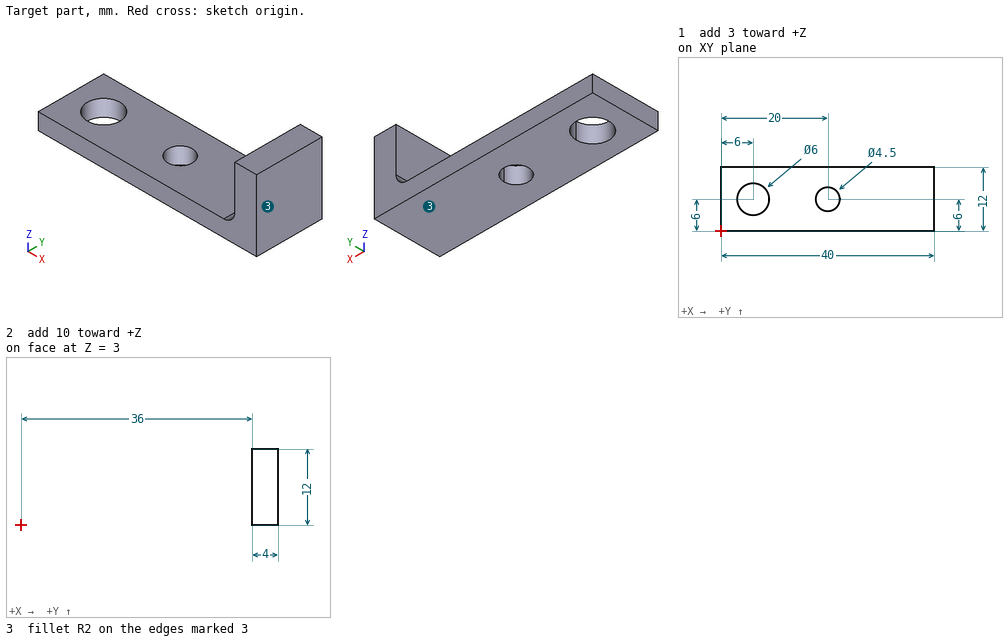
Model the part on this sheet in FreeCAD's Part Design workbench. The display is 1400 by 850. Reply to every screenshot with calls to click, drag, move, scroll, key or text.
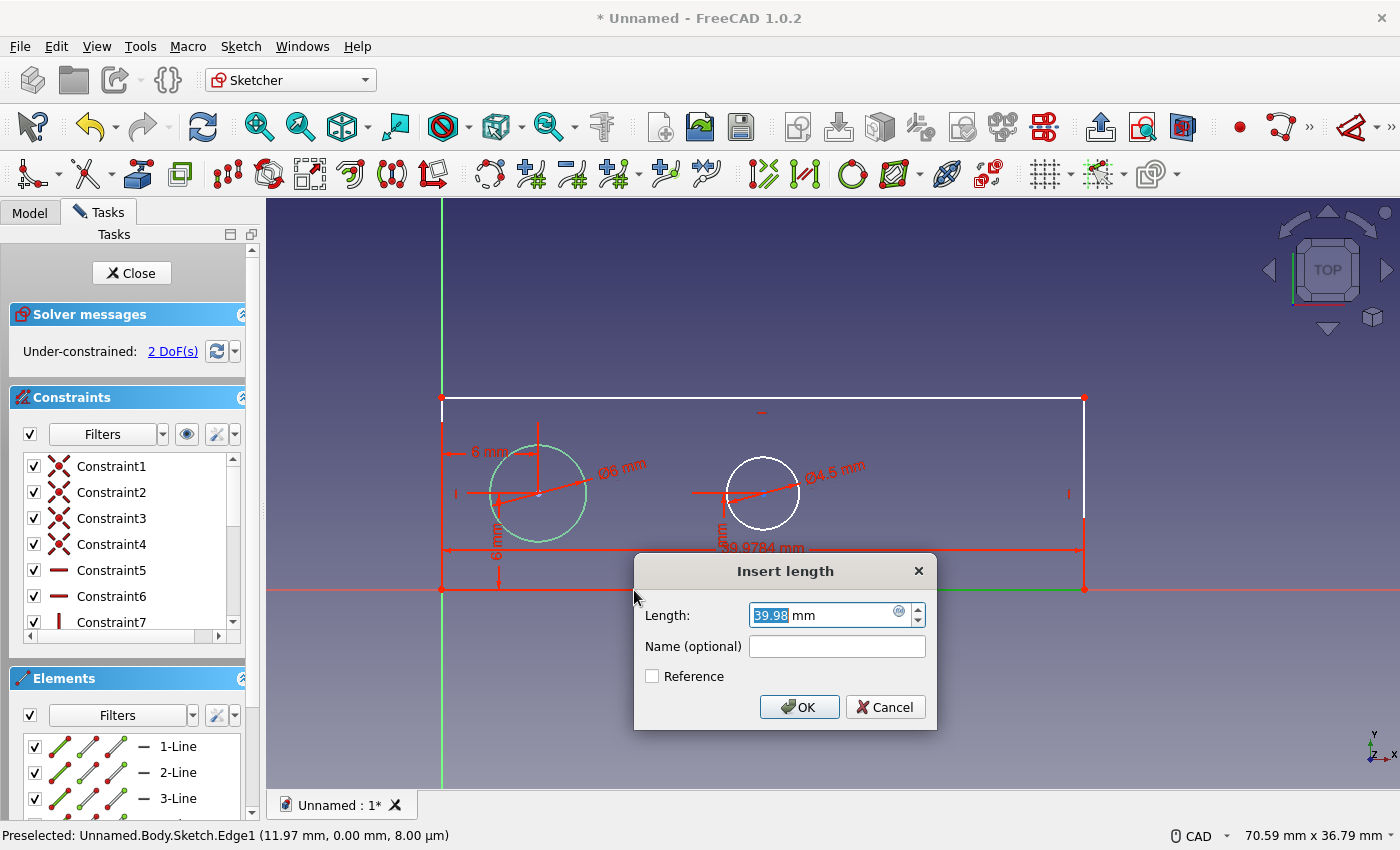
text(40)
key(Return)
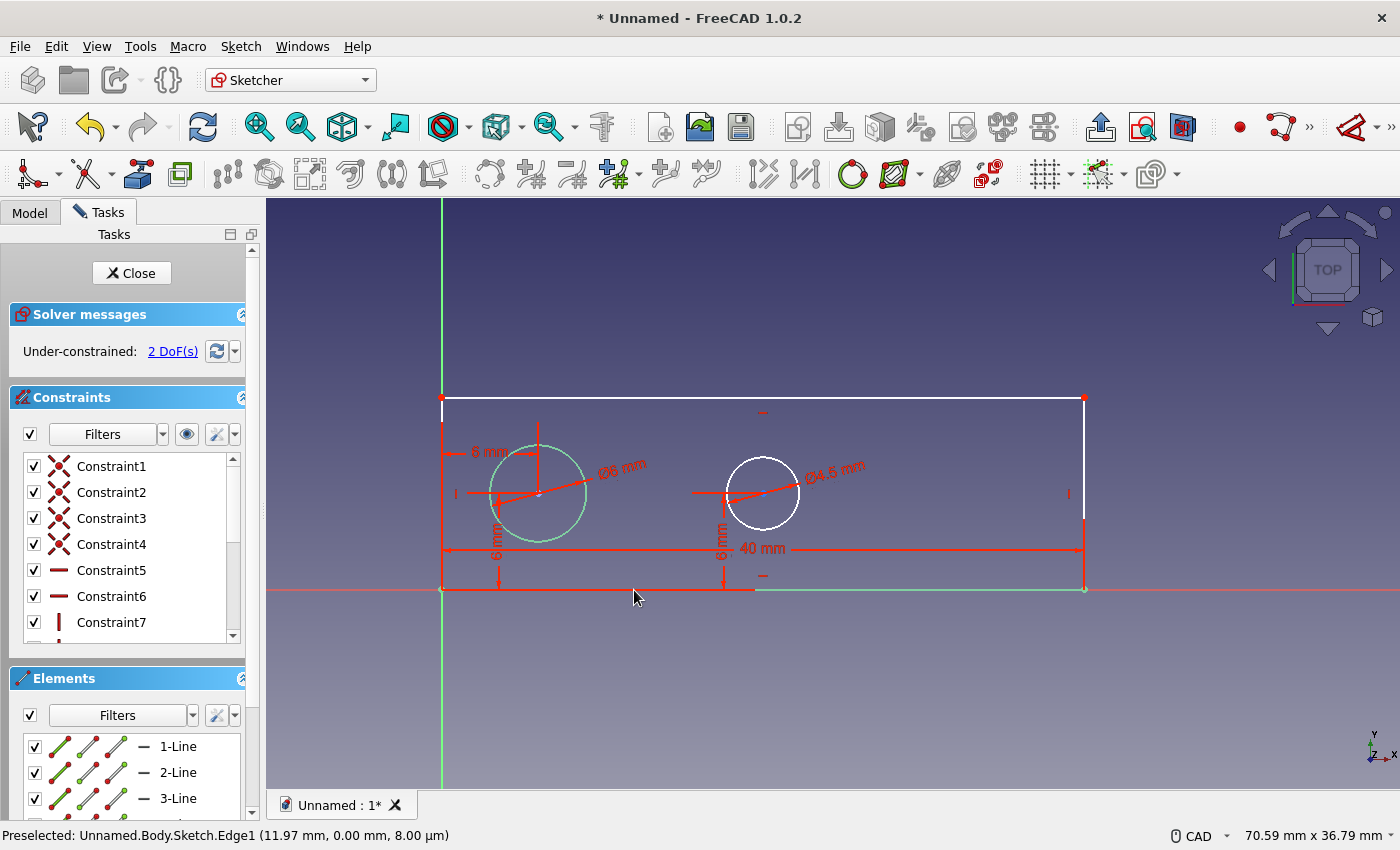
click(1084, 532)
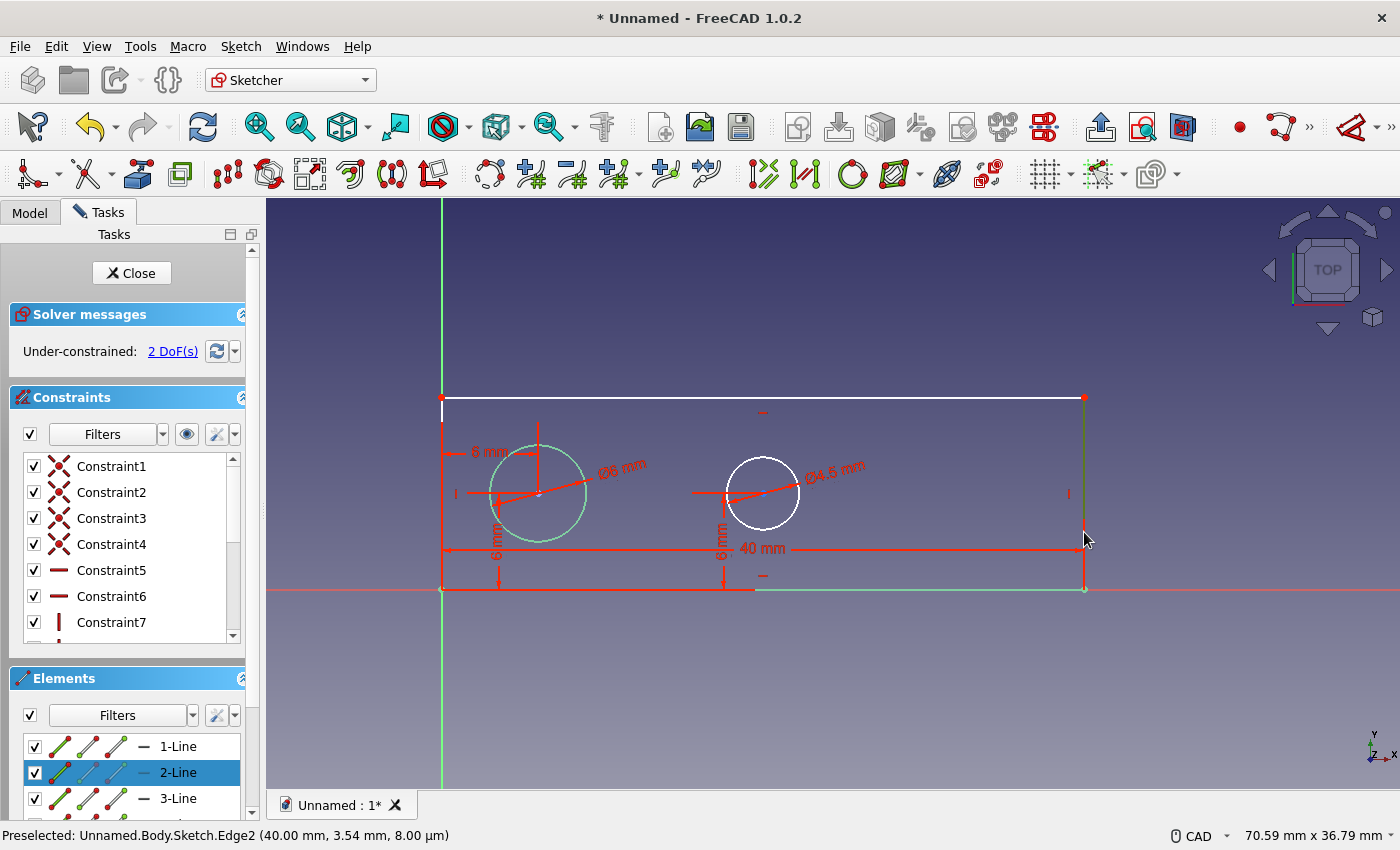
click(1376, 128)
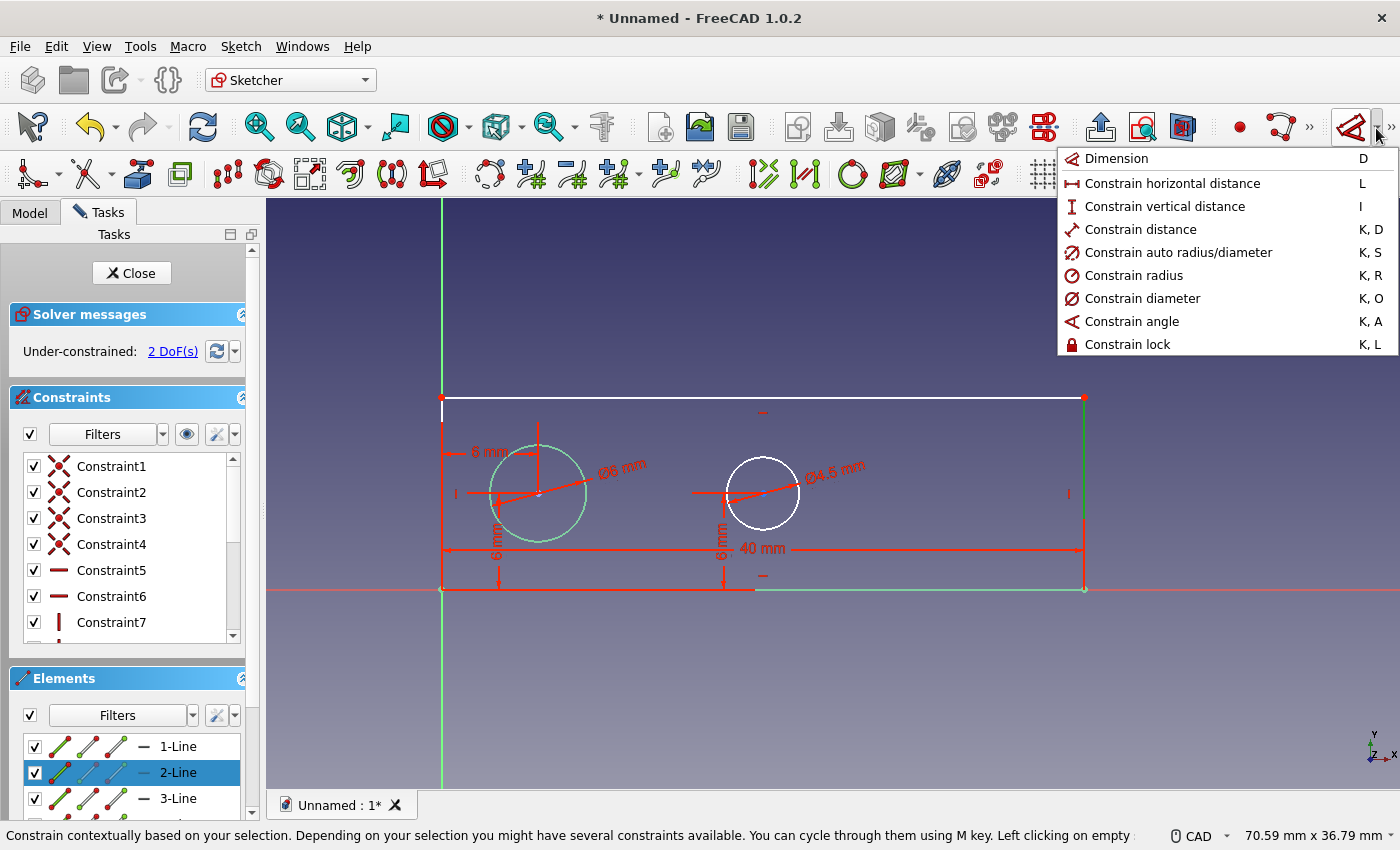
click(1228, 206)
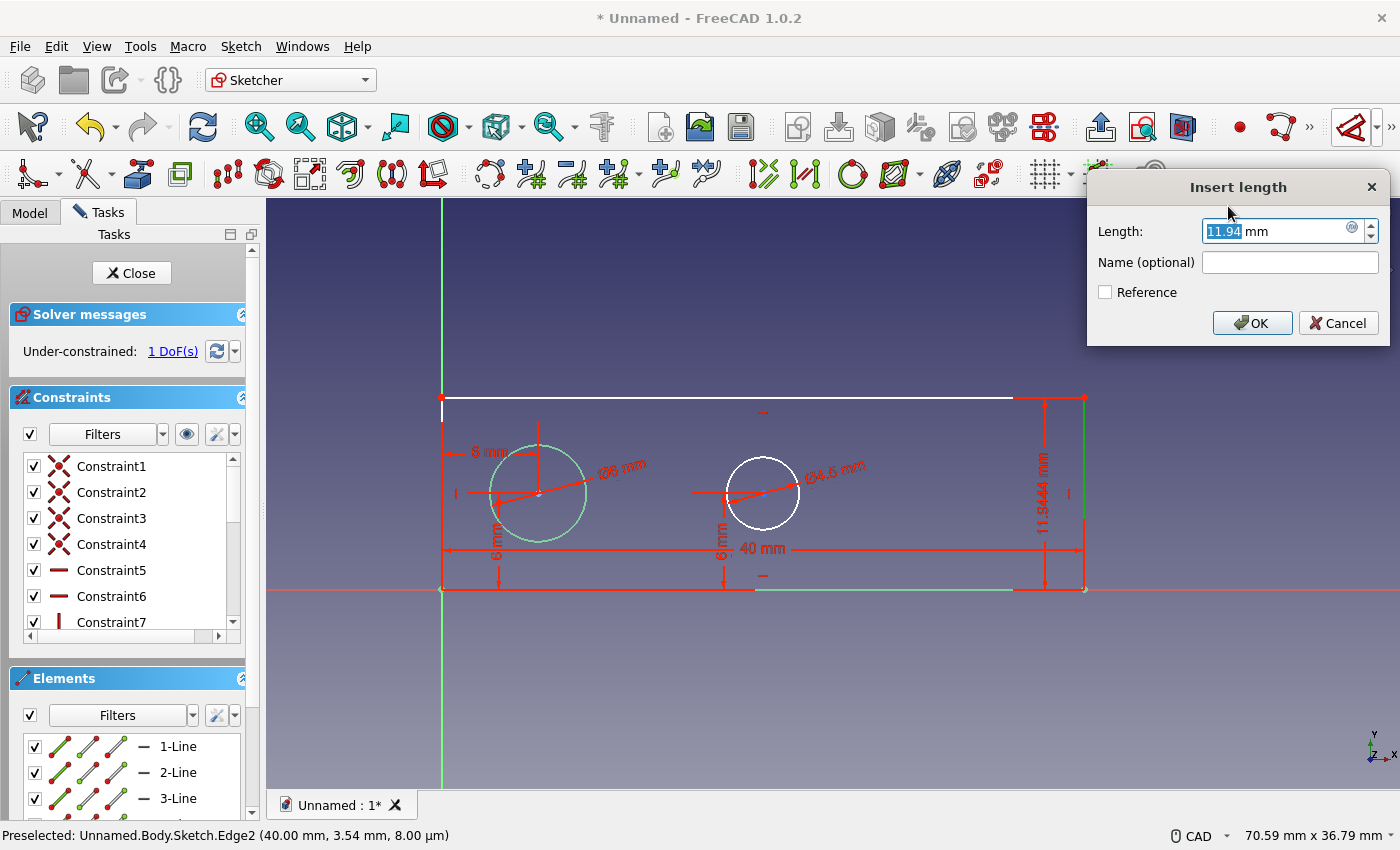
text(12)
key(Return)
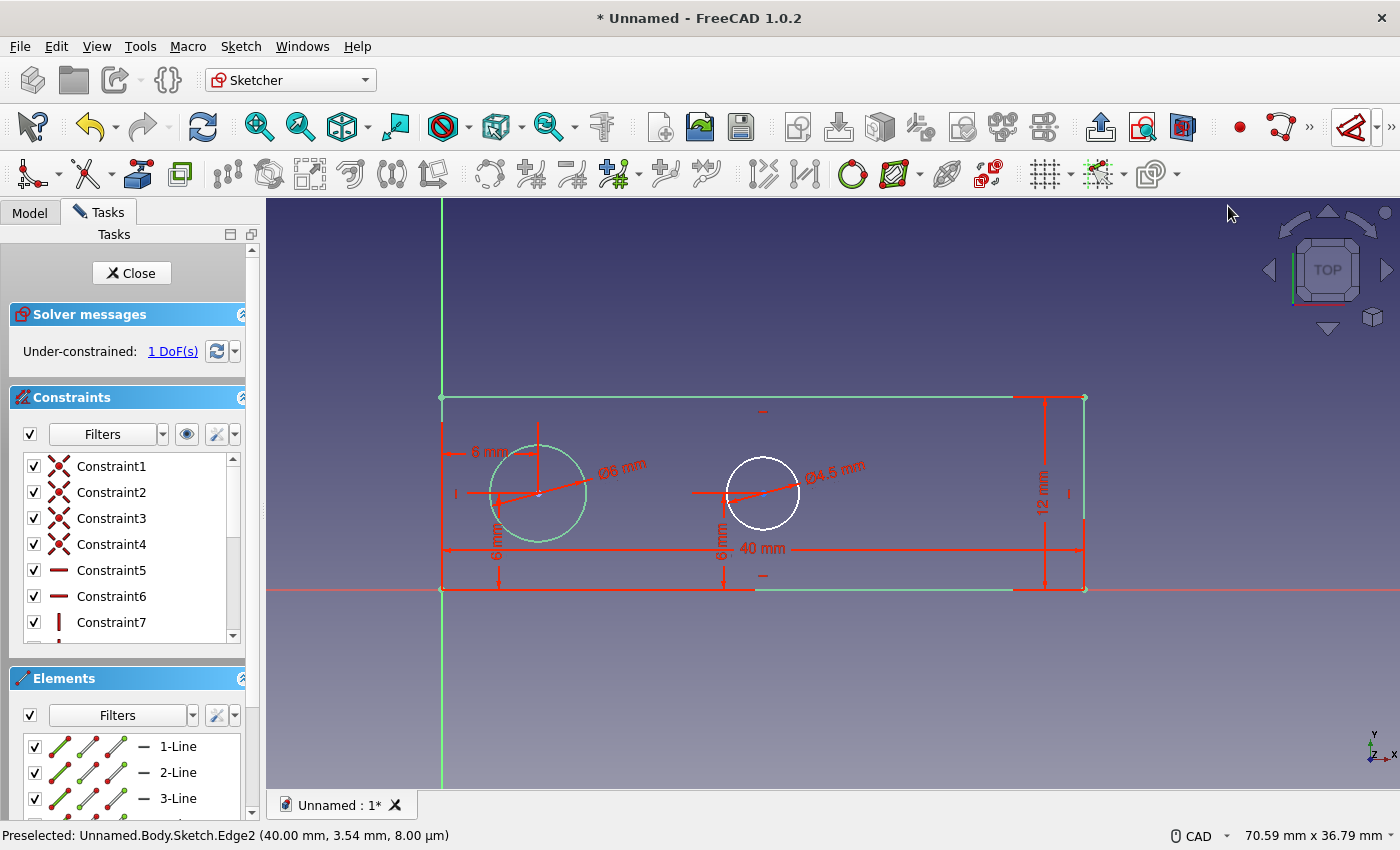
click(763, 493)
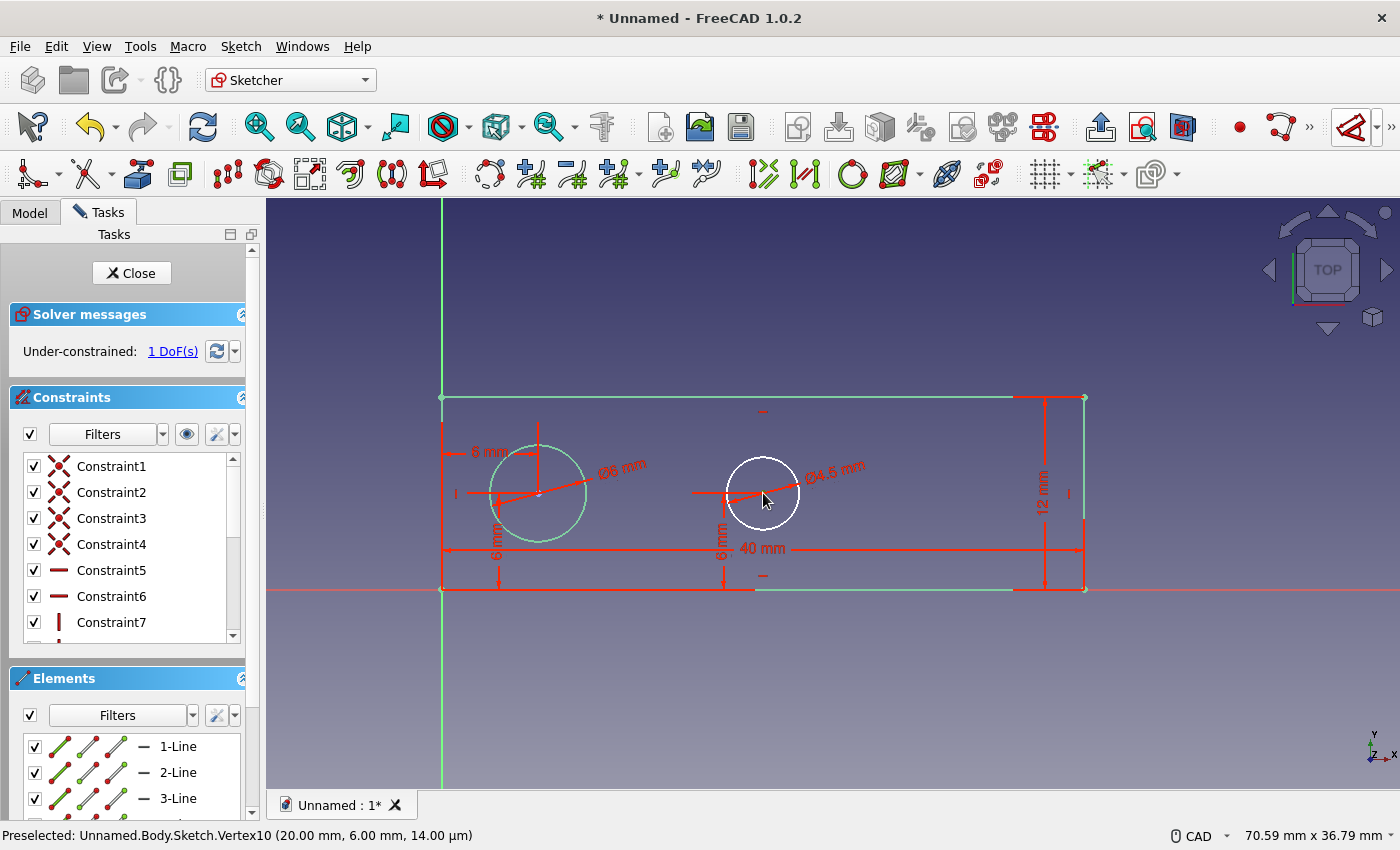
click(1376, 128)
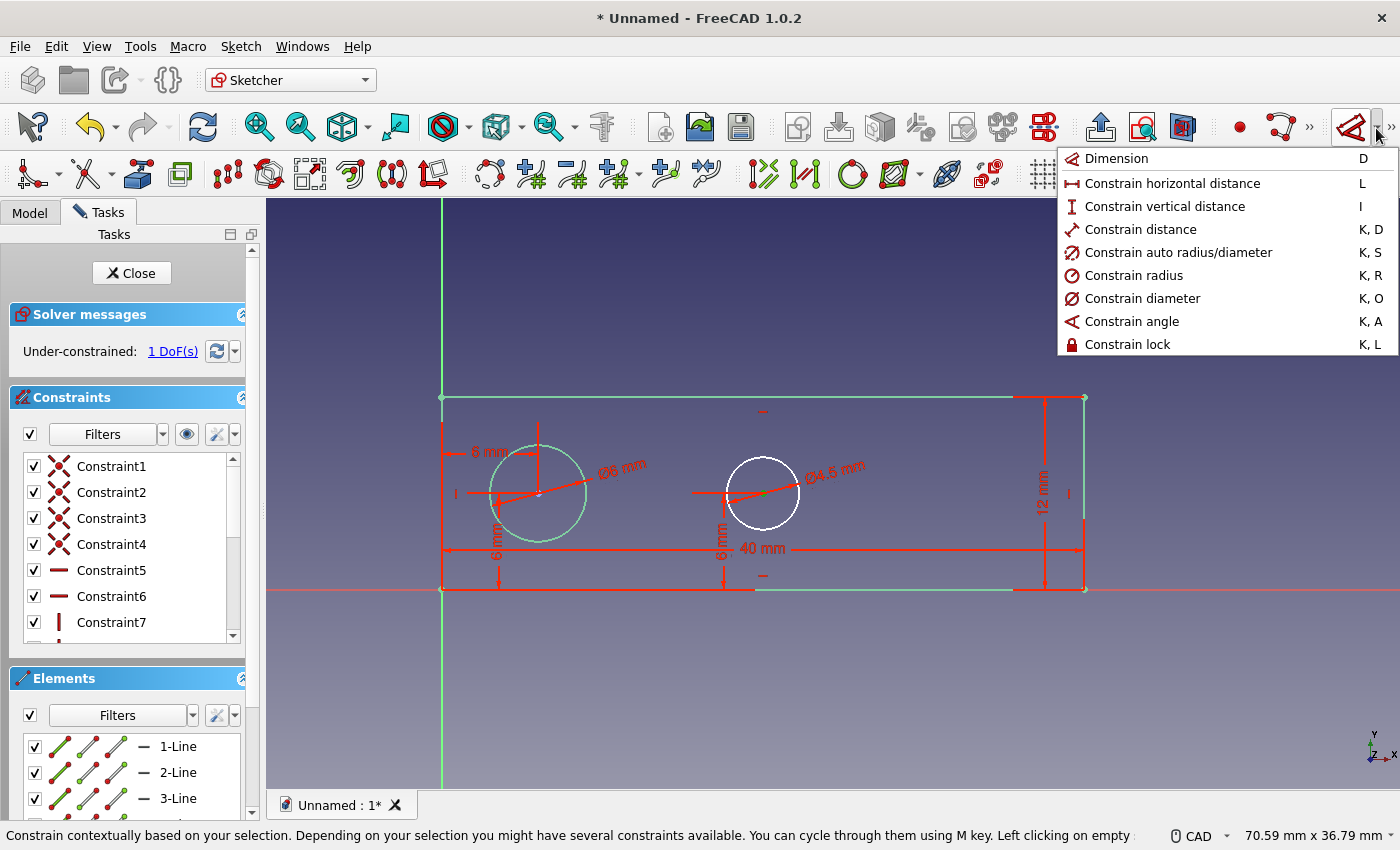
click(1228, 184)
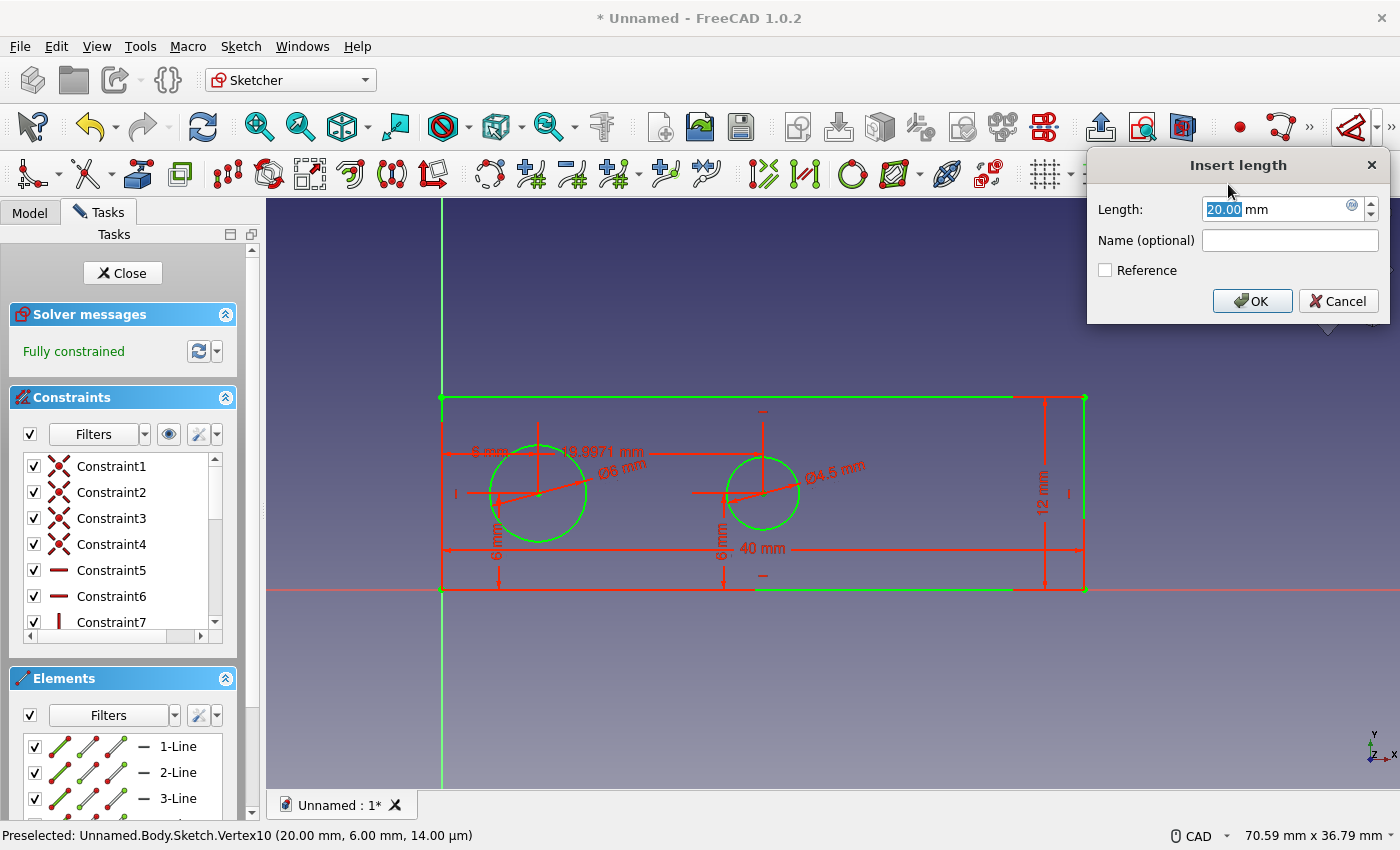
text(20)
key(Return)